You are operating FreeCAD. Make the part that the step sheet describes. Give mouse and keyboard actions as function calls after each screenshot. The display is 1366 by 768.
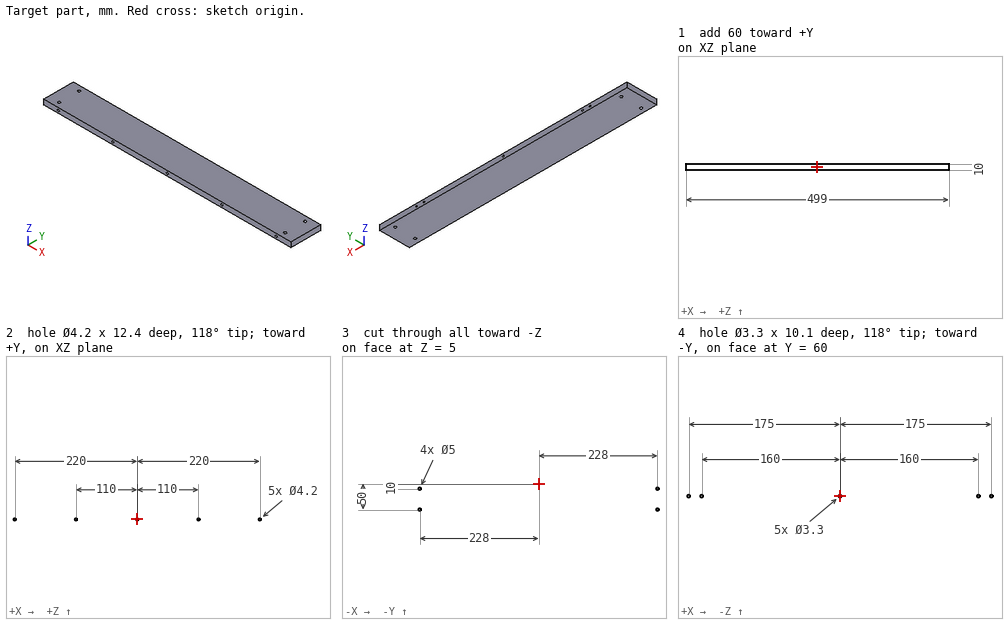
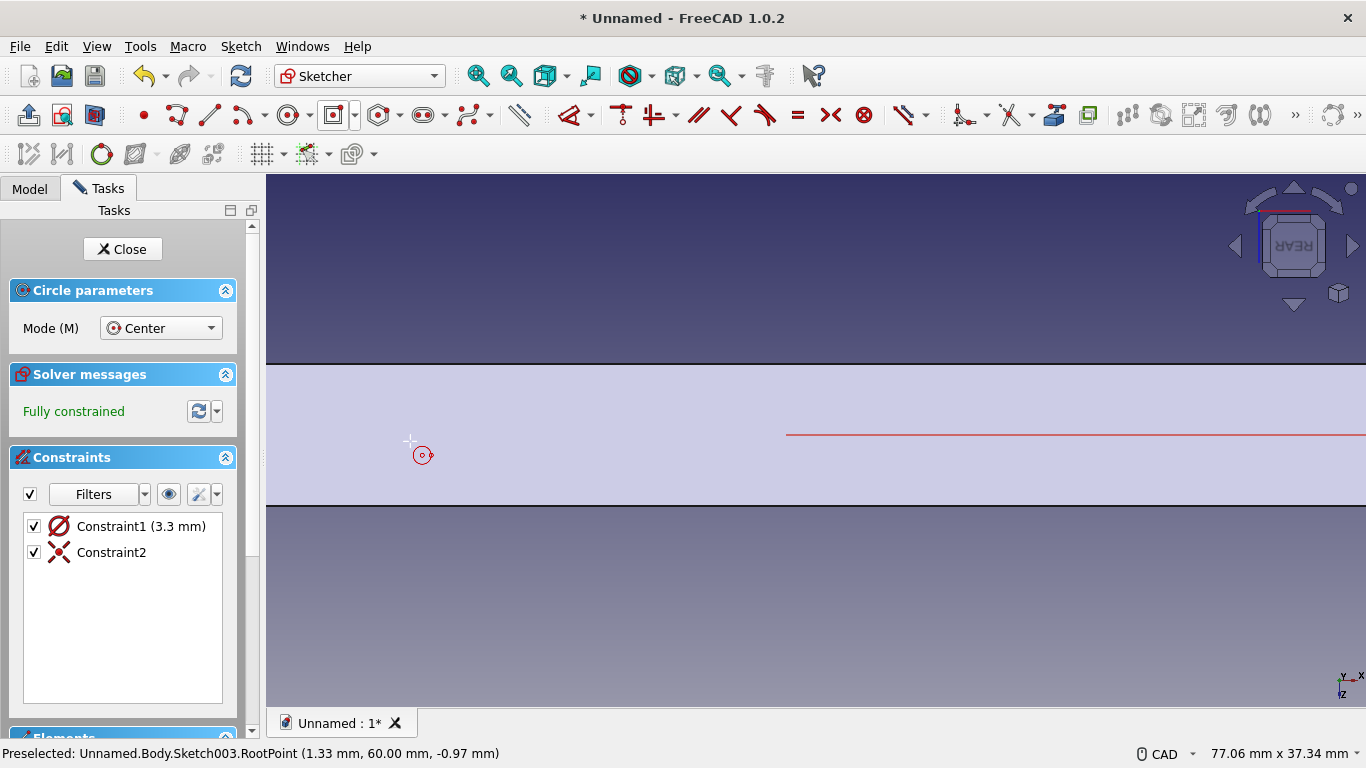
scroll(410, 441, down, 10)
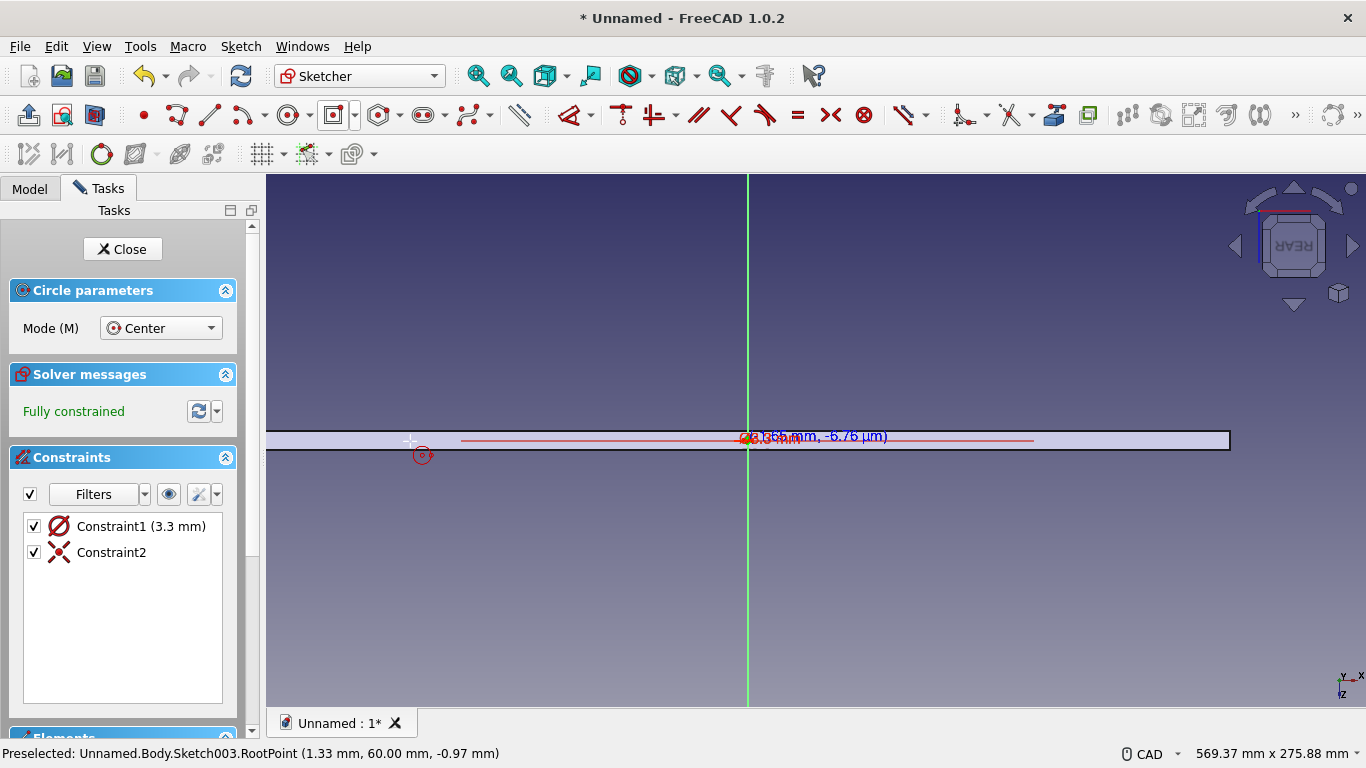
click(410, 441)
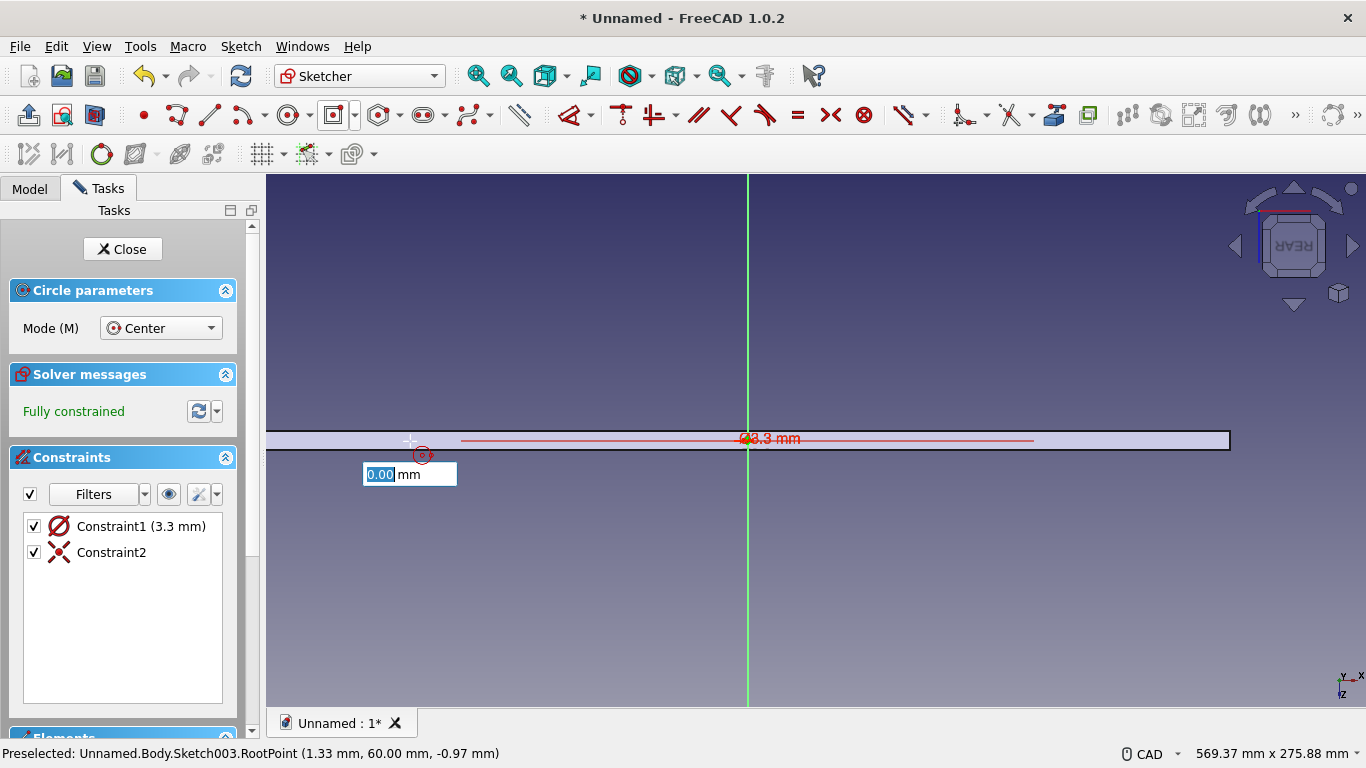
scroll(409, 444, up, 9)
move(405, 439)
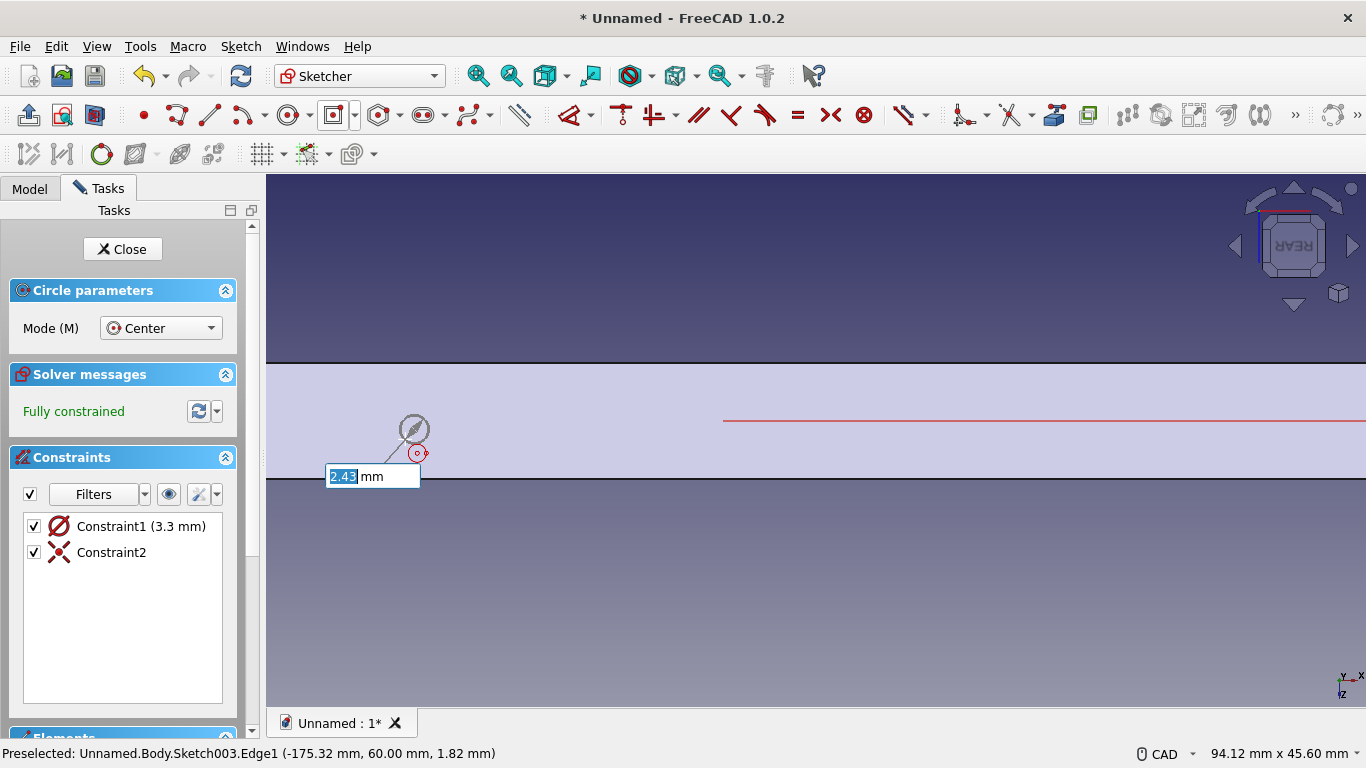
text(3.3)
key(Return)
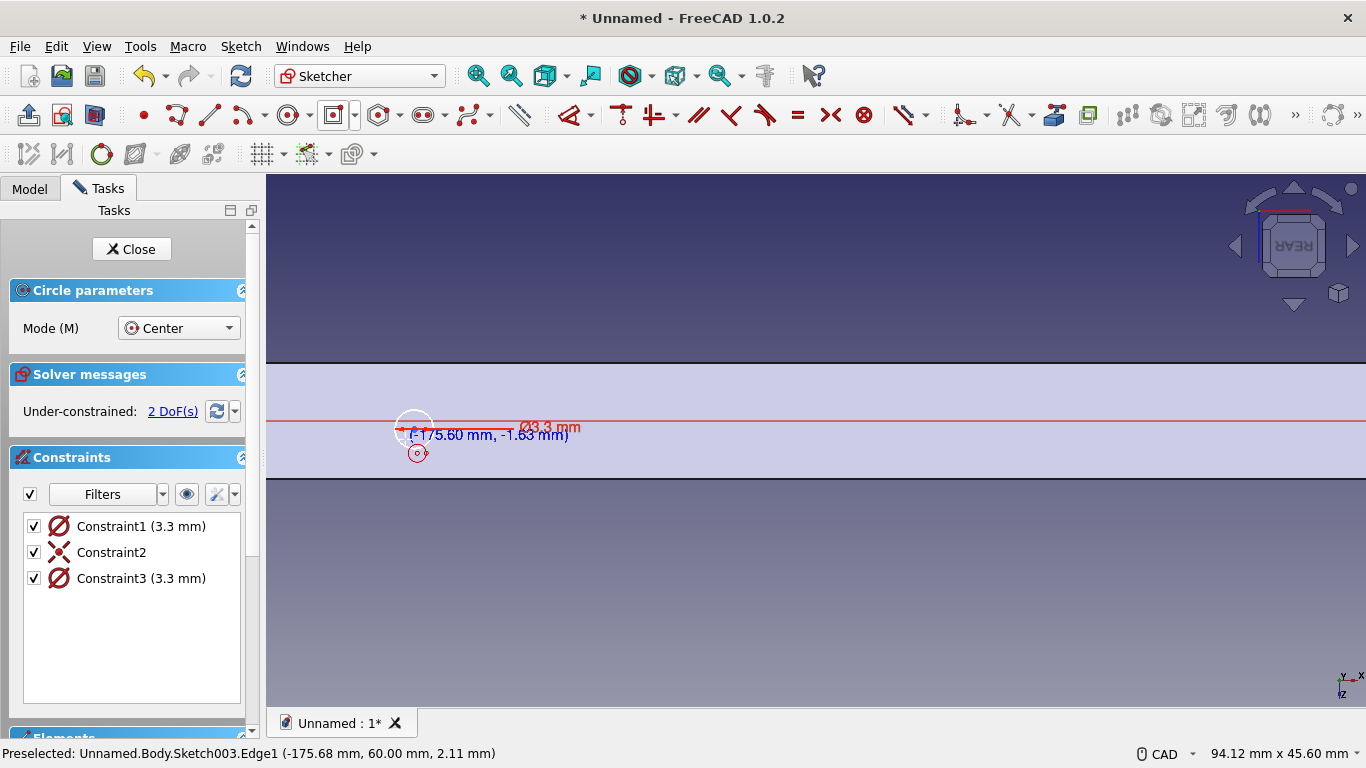
scroll(409, 444, down, 9)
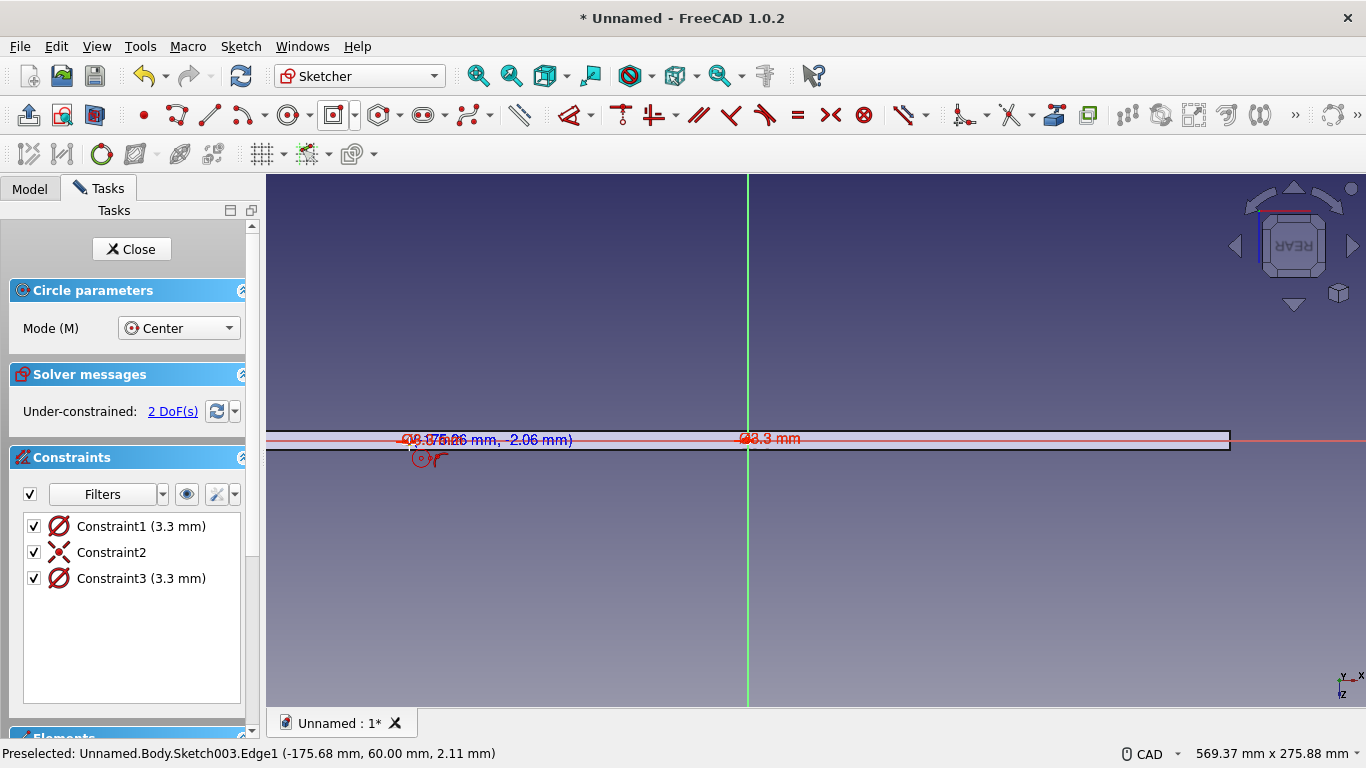
scroll(1086, 441, up, 10)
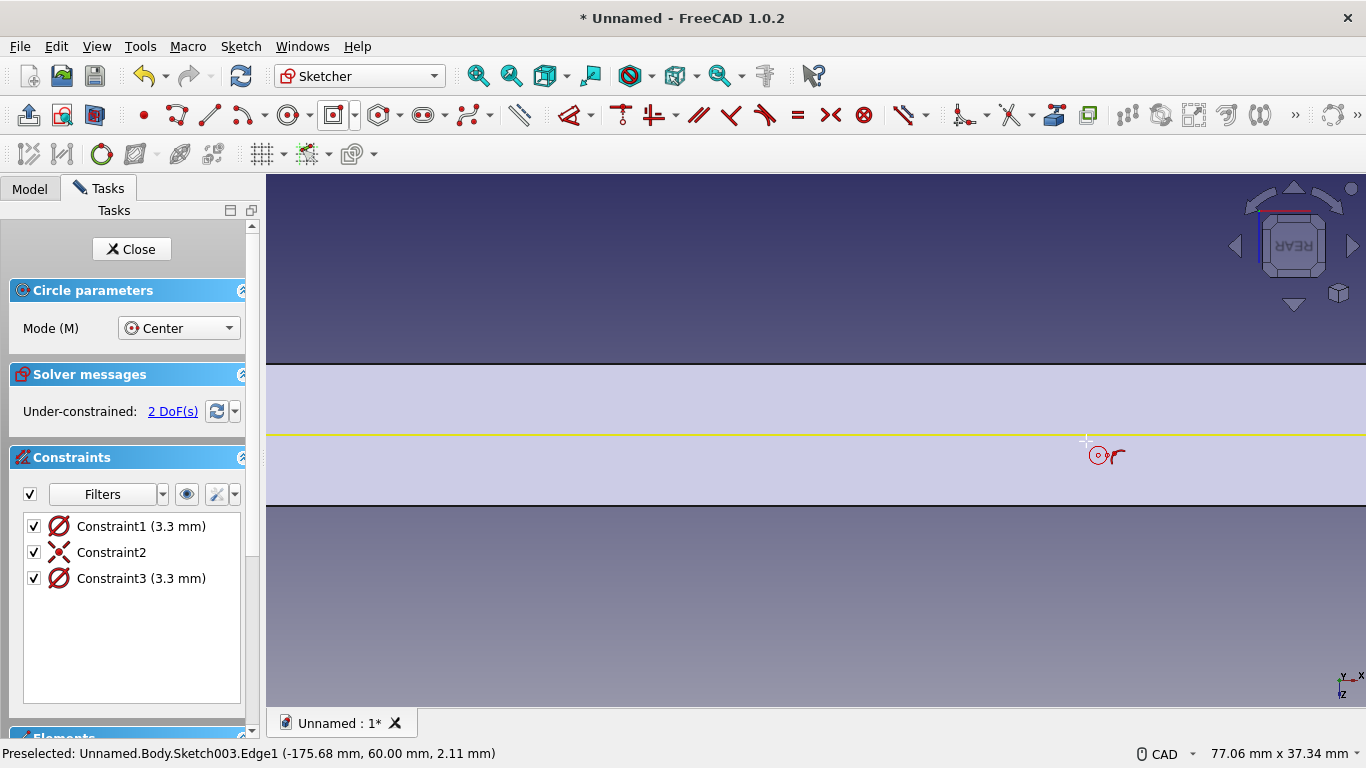
scroll(1087, 441, down, 10)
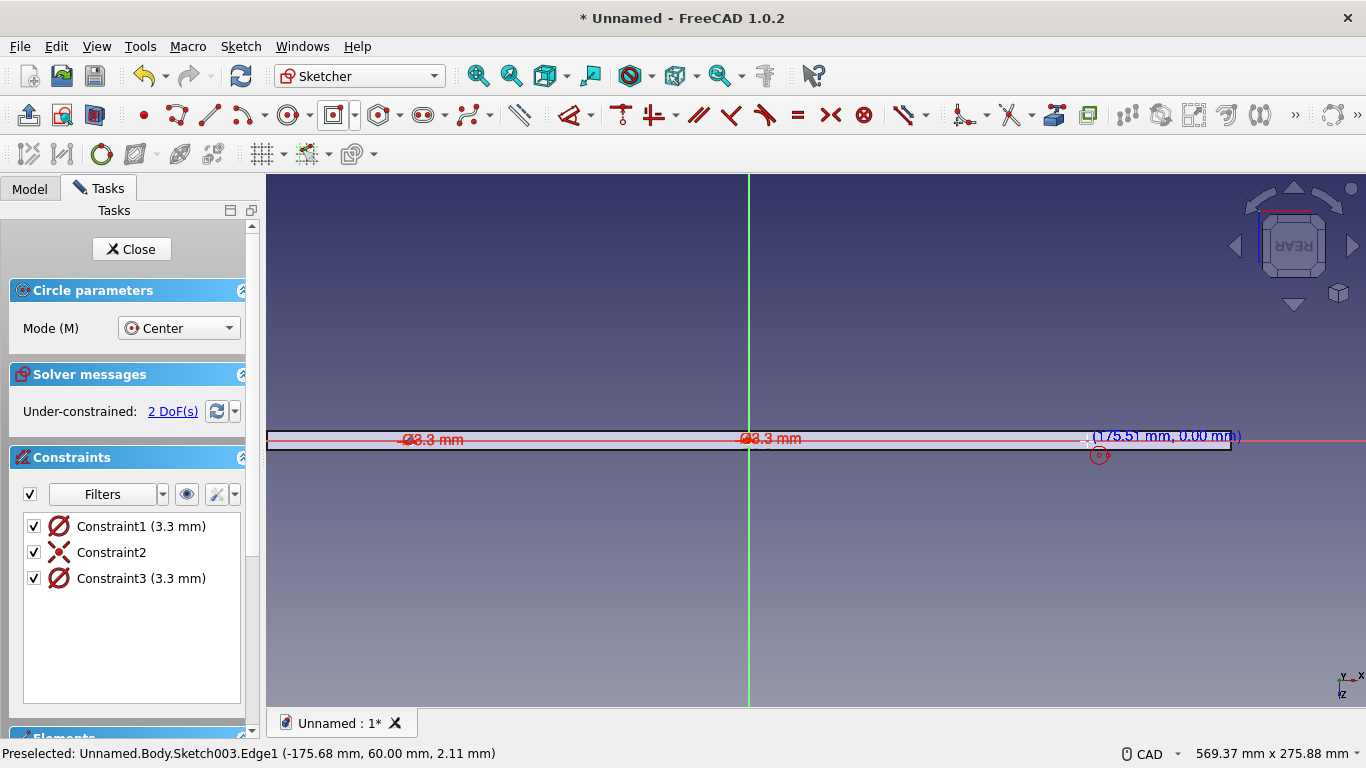
click(1087, 441)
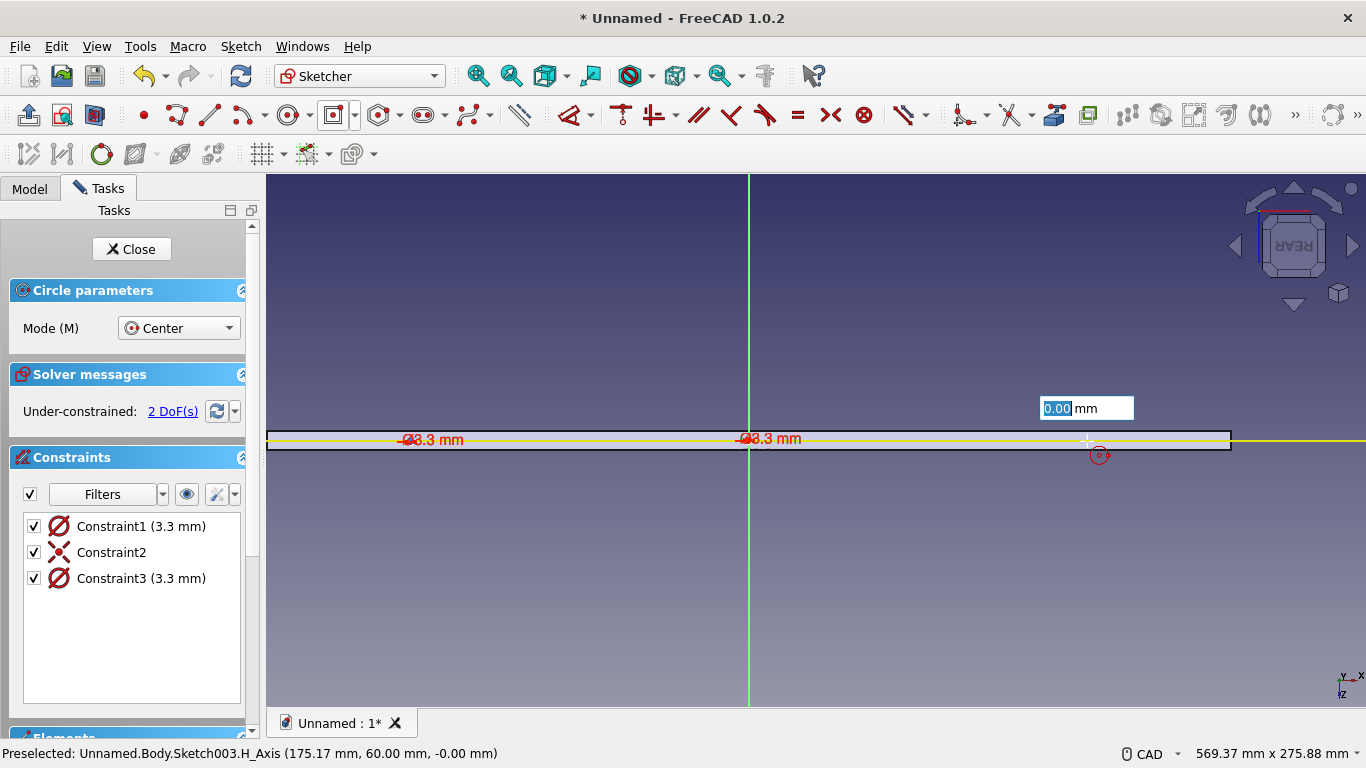
scroll(1086, 444, up, 9)
move(1080, 439)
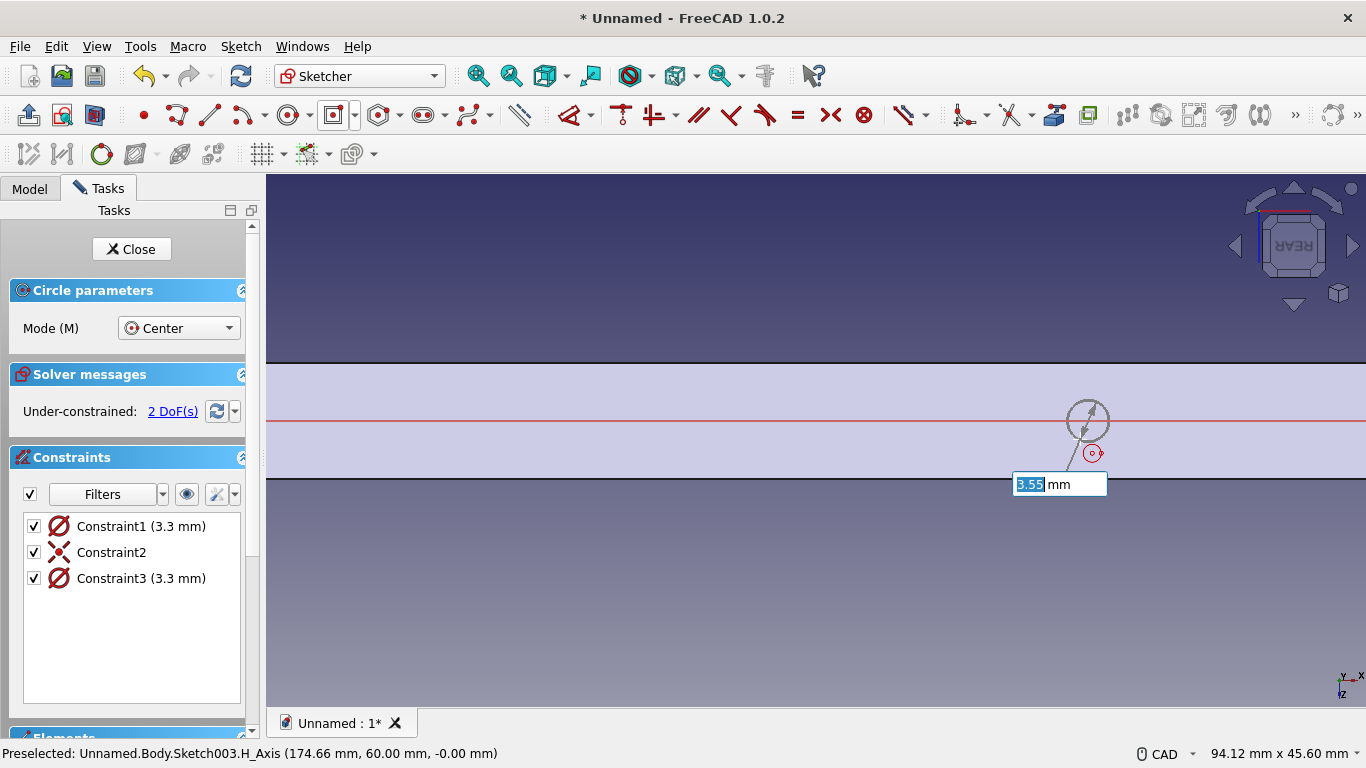
text(3.3)
key(Return)